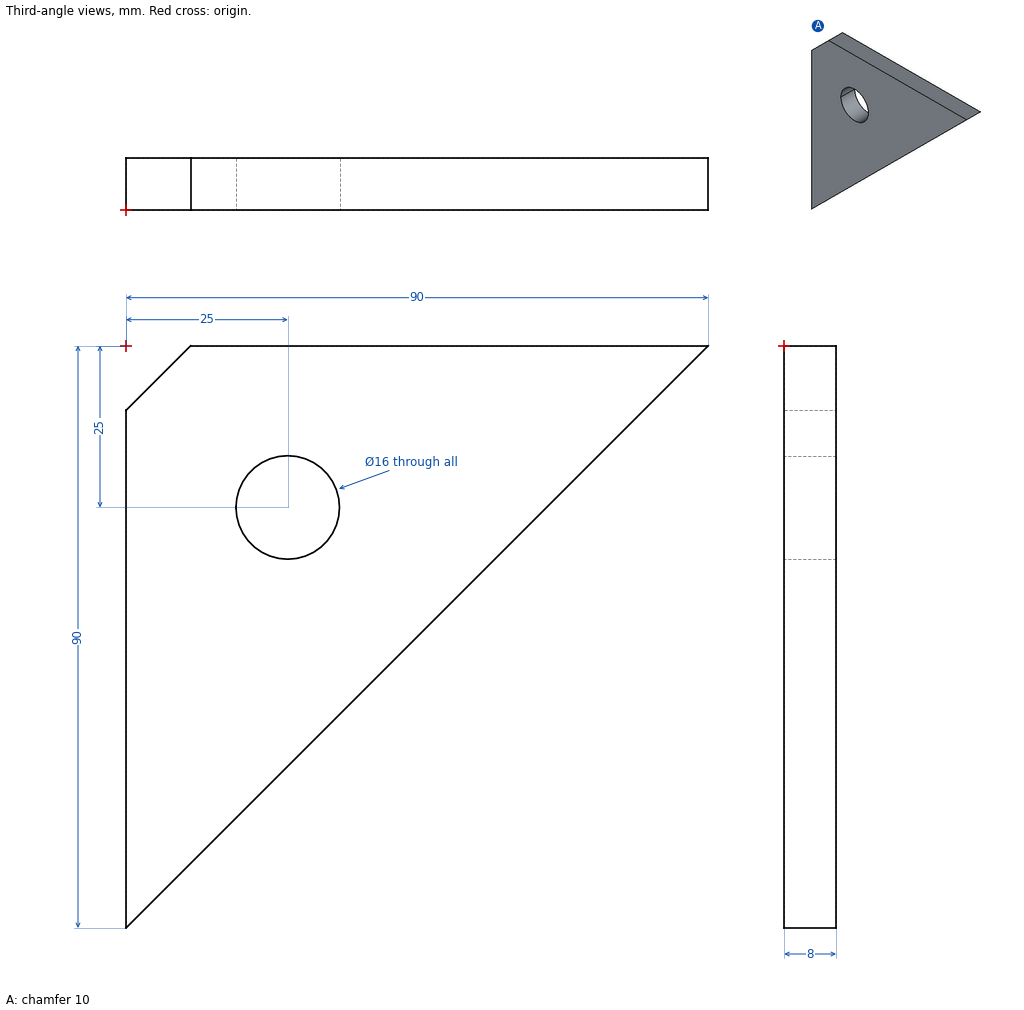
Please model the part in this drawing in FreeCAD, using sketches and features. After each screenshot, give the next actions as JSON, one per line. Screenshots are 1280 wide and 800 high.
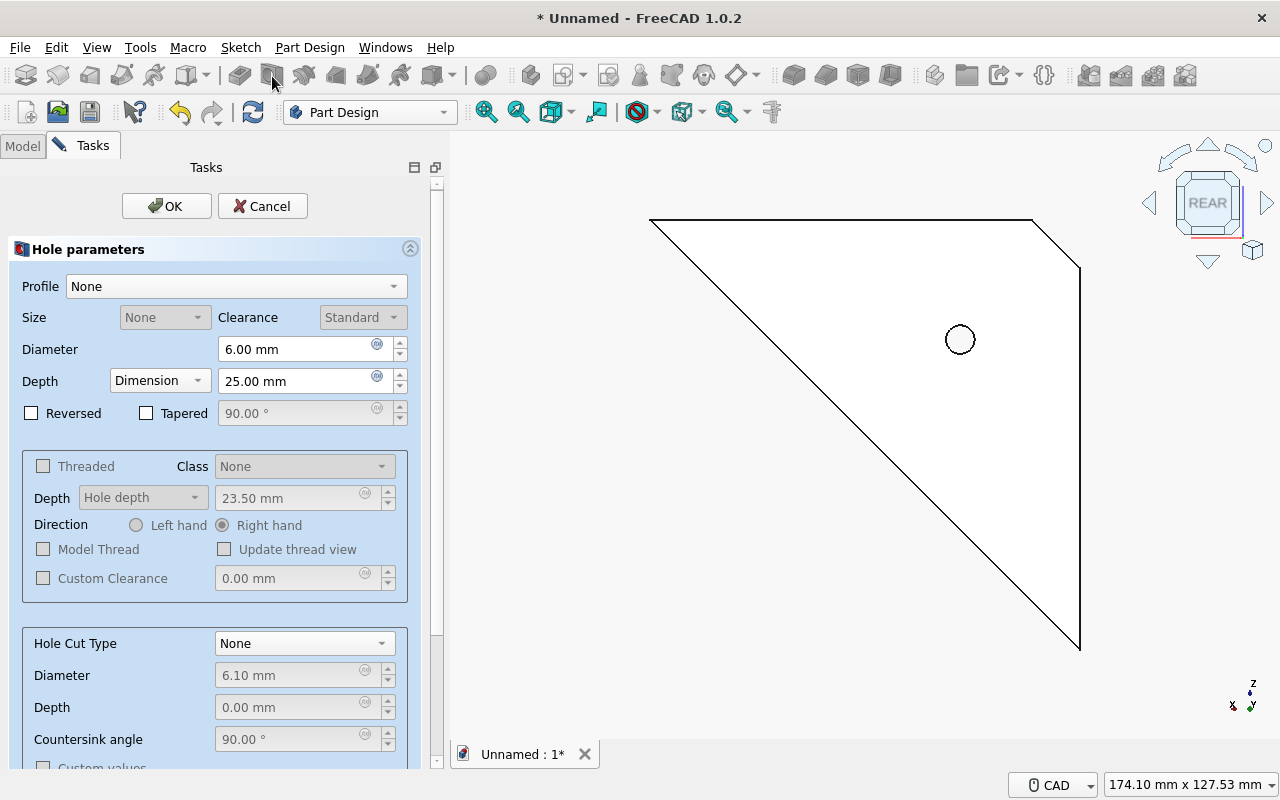
{"action": "triple_click", "coordinate": [305, 349]}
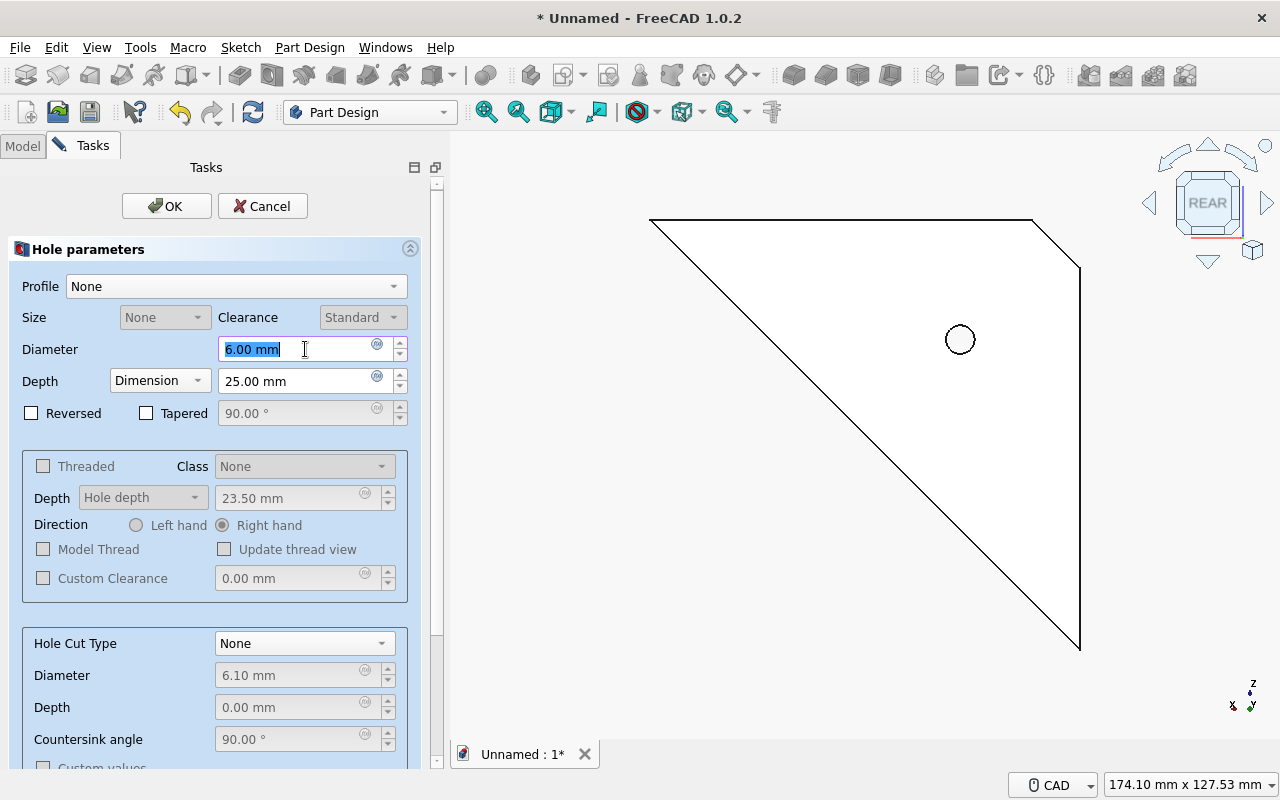
{"action": "type", "text": "16"}
{"action": "key", "text": "Tab"}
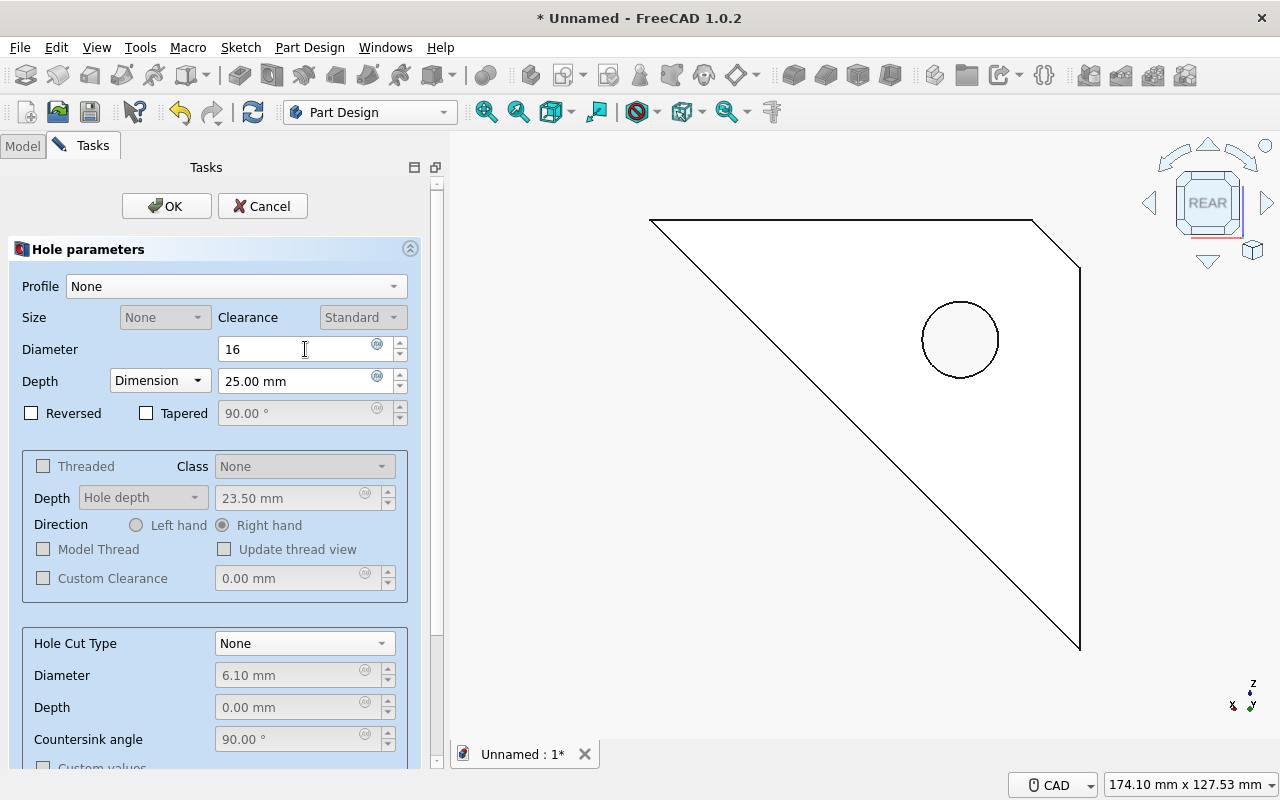
{"action": "left_click", "coordinate": [161, 380]}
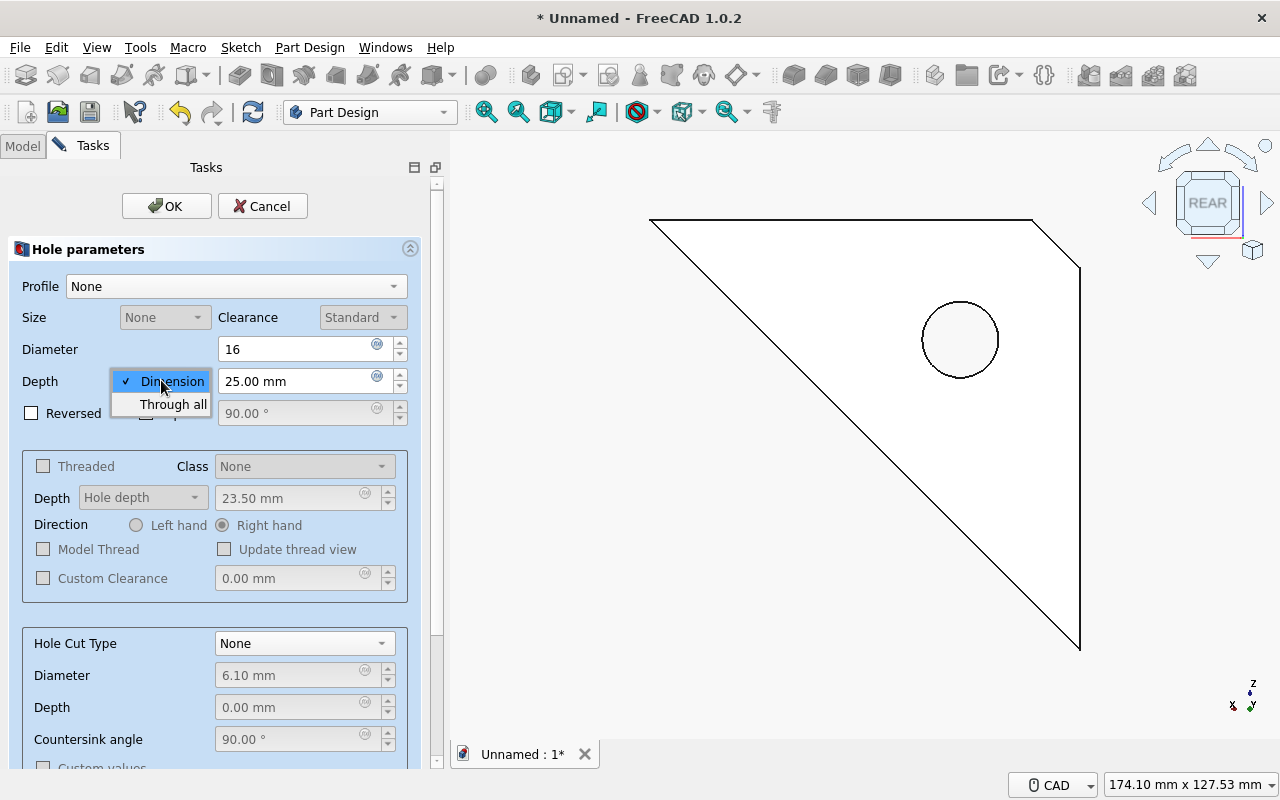
{"action": "left_click", "coordinate": [160, 404]}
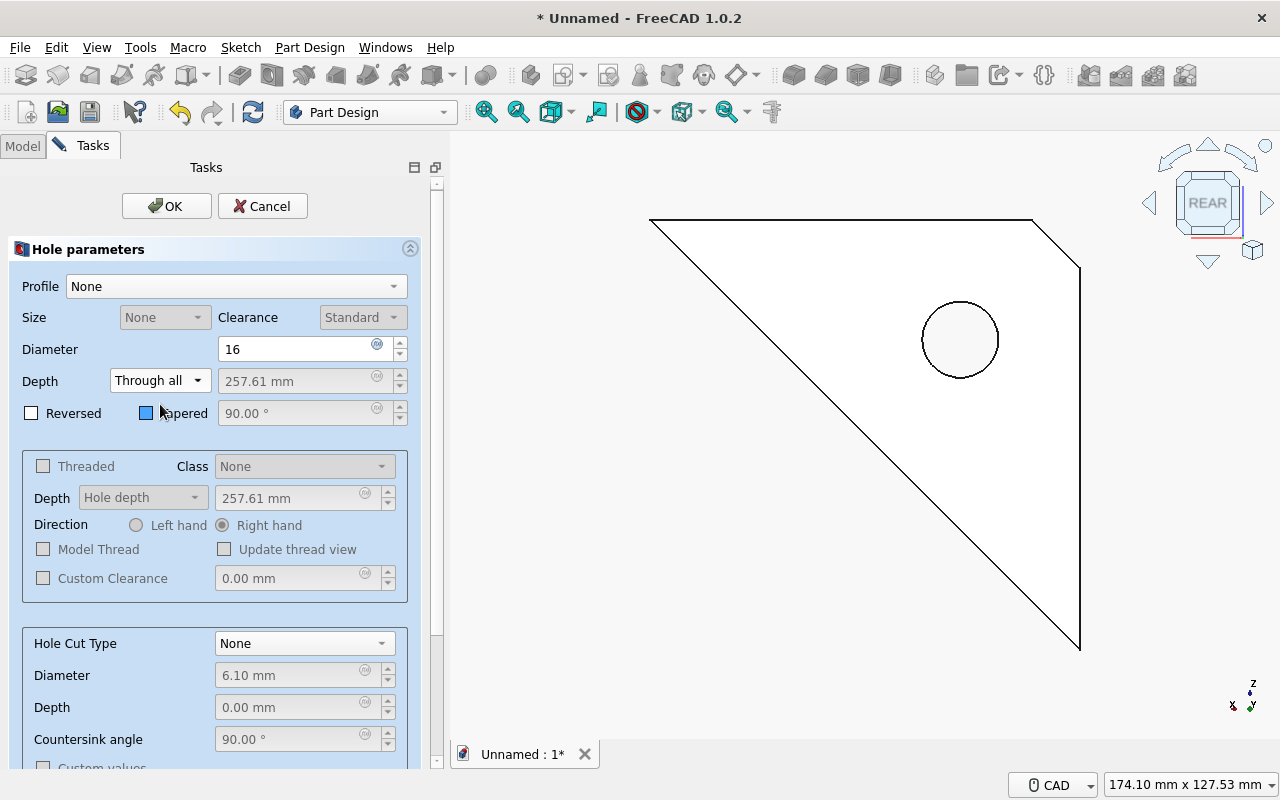
{"action": "left_click", "coordinate": [167, 206]}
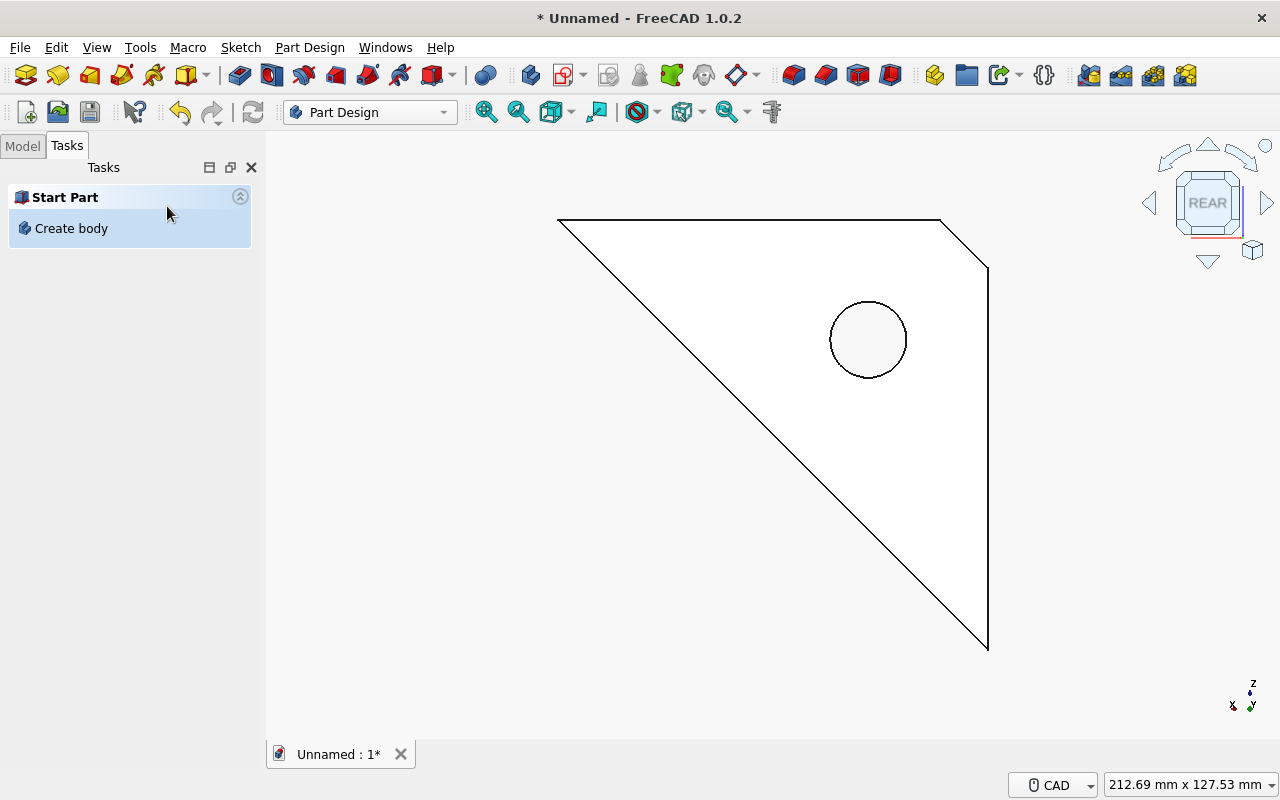
{"action": "key", "text": "0"}